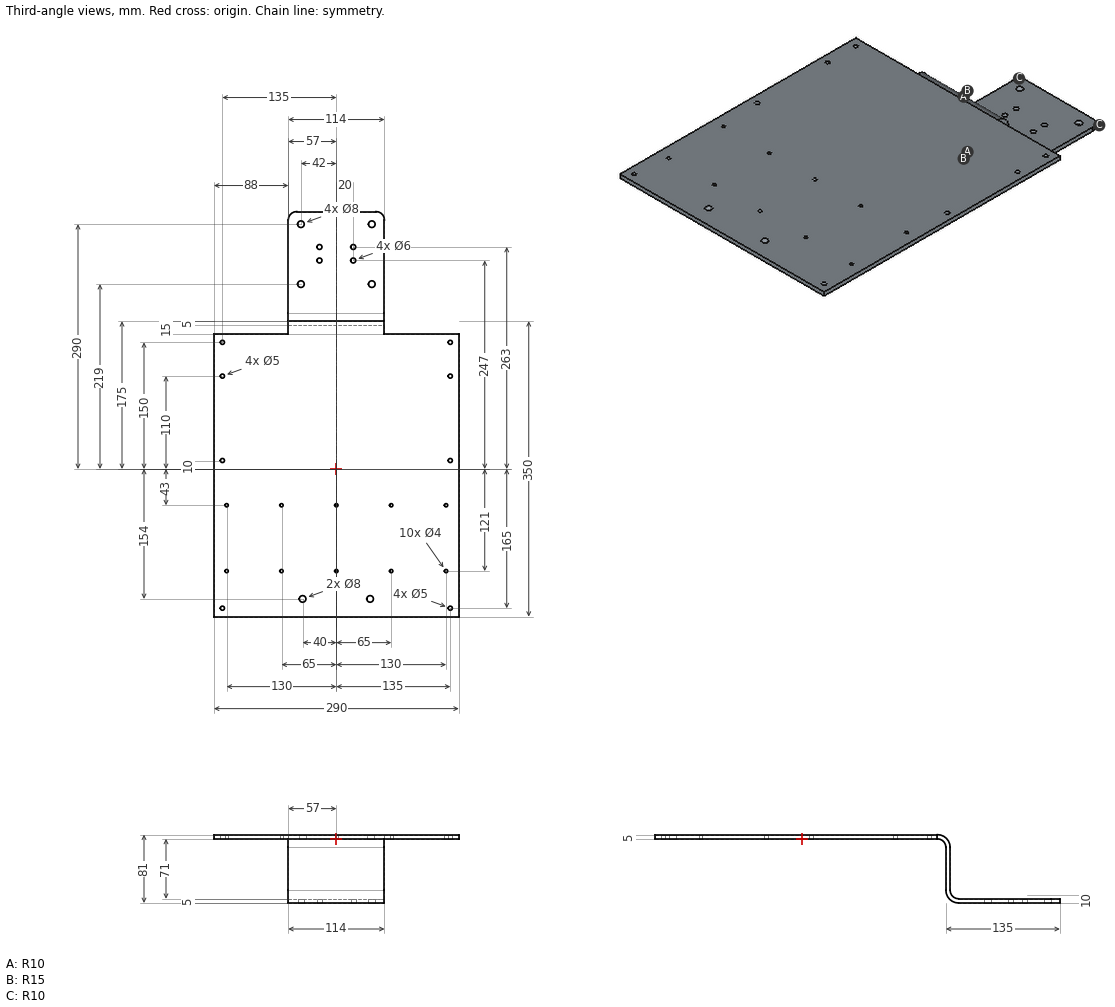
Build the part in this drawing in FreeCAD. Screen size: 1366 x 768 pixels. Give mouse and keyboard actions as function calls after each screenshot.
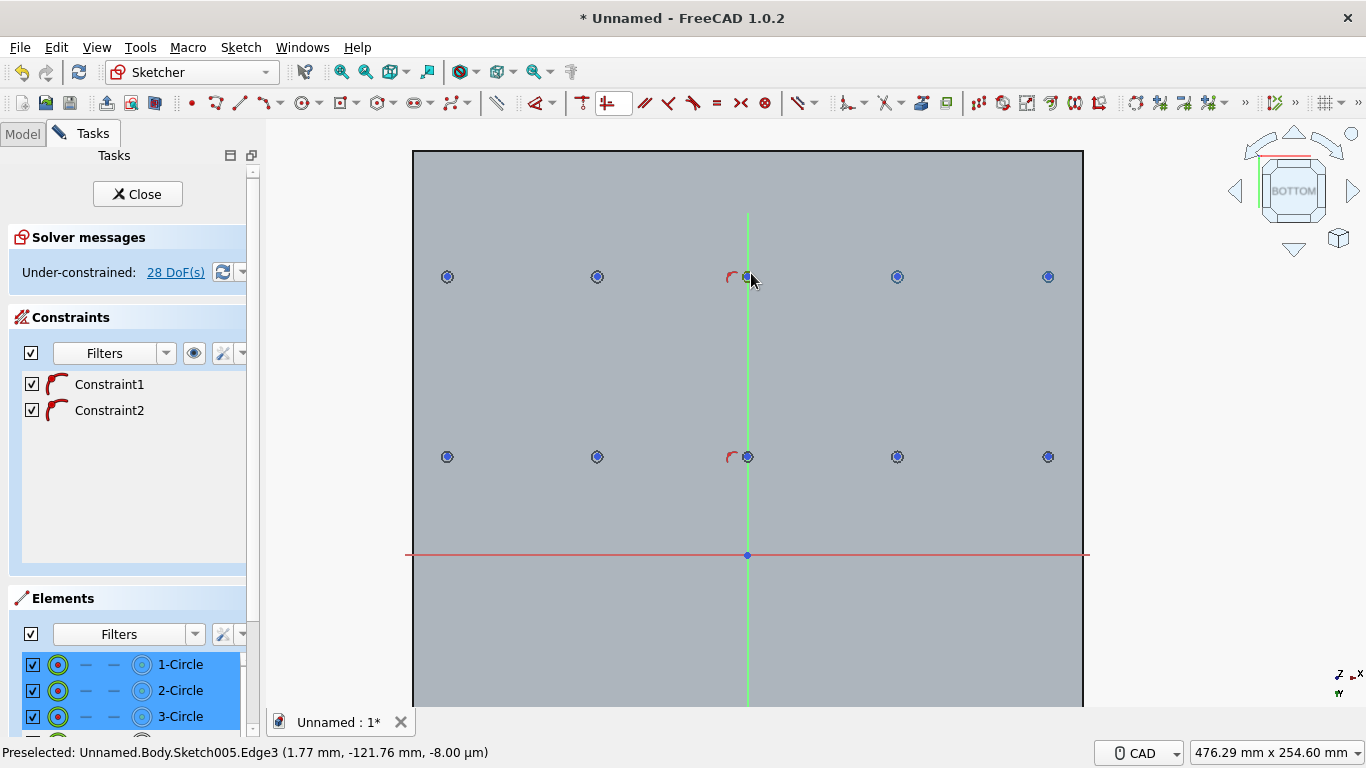
scroll(601, 273, up, 5)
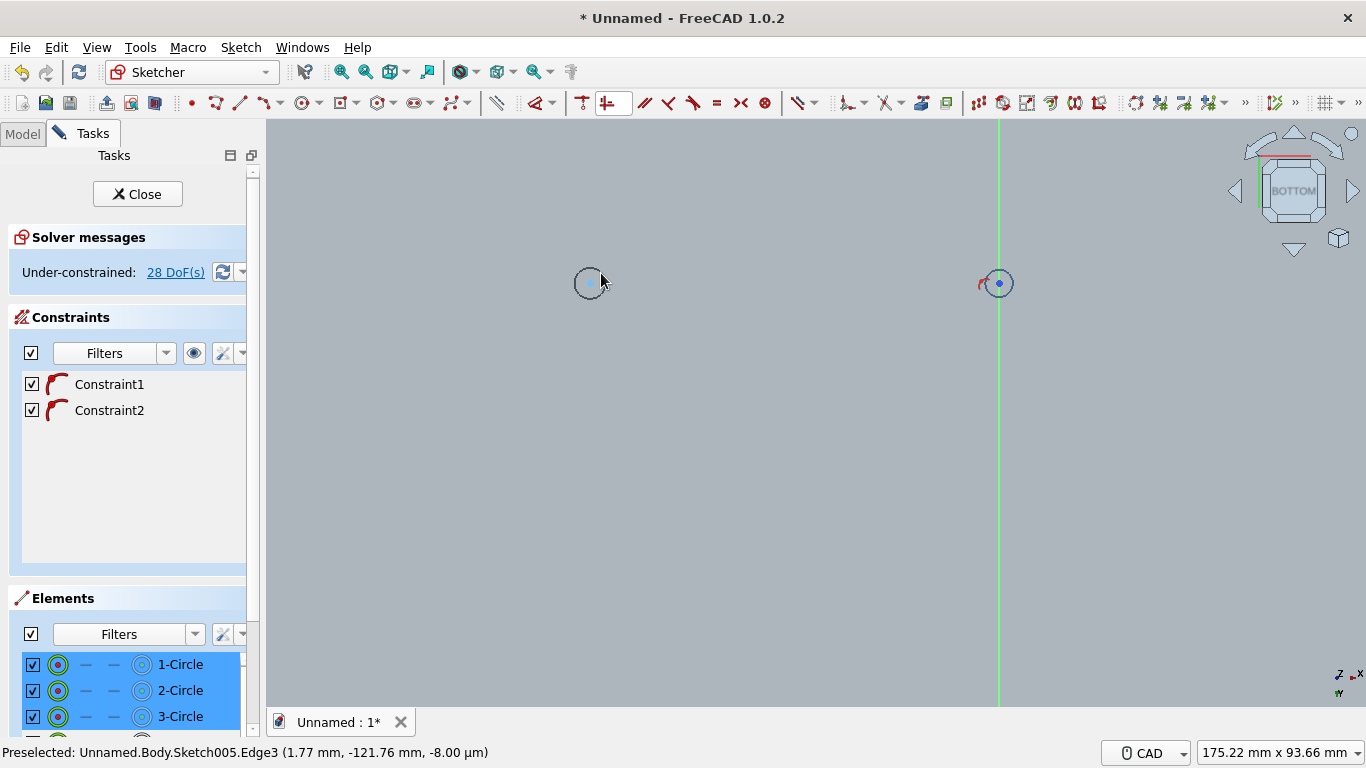
click(601, 272)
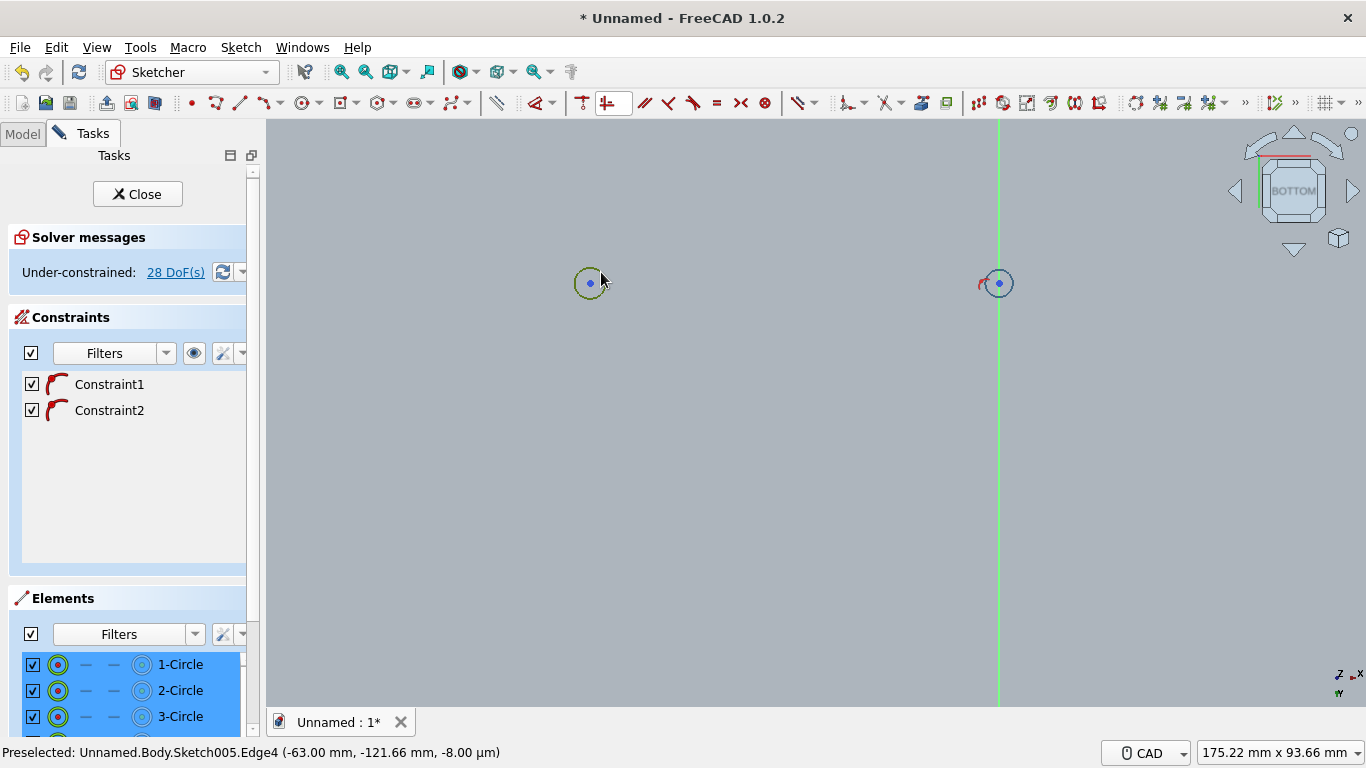
scroll(601, 273, down, 5)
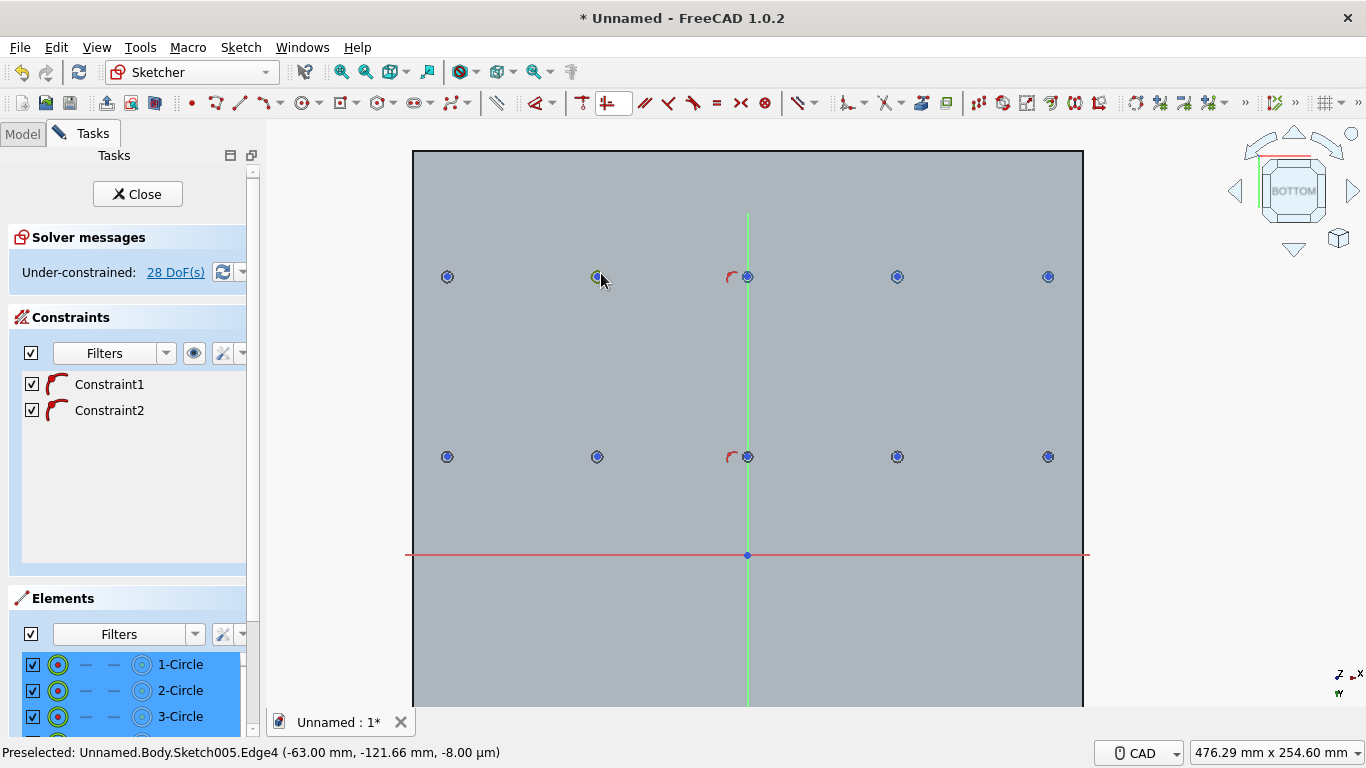
scroll(451, 273, up, 5)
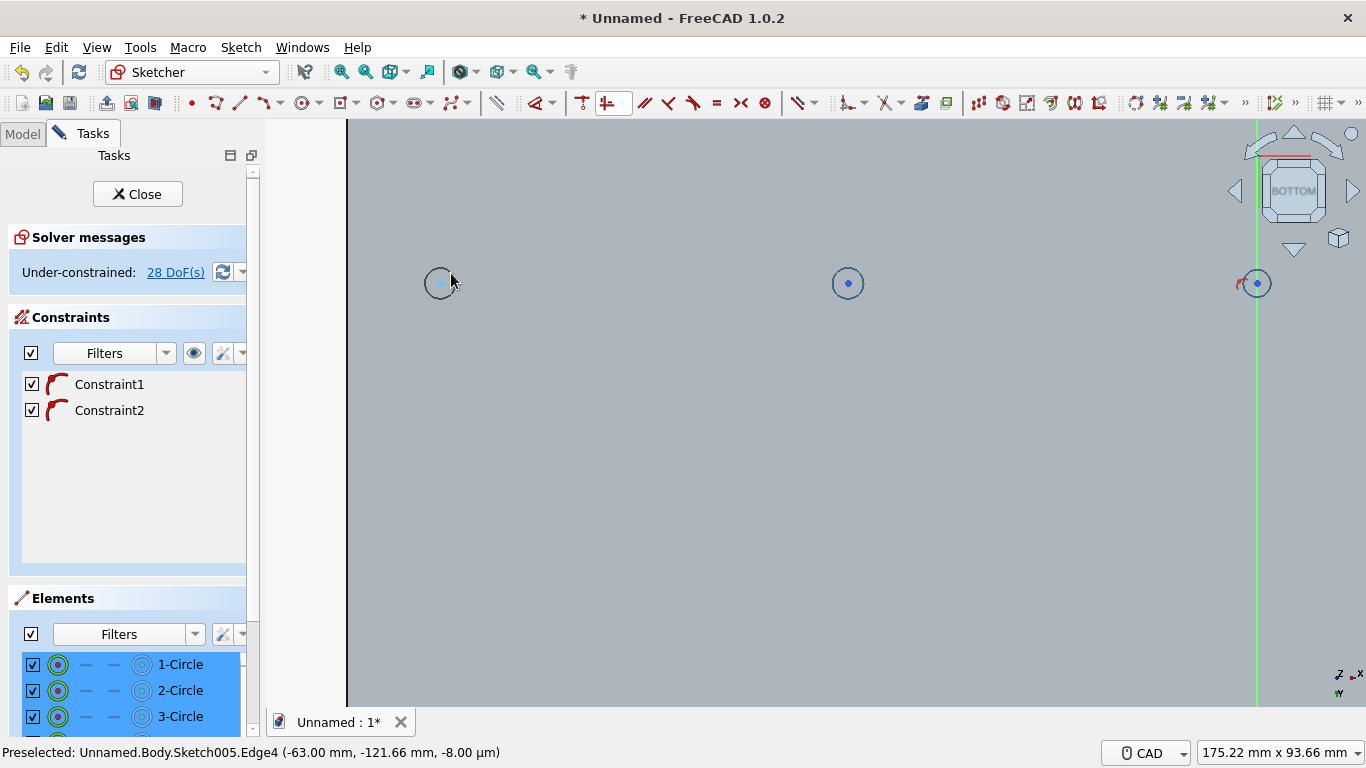
click(451, 273)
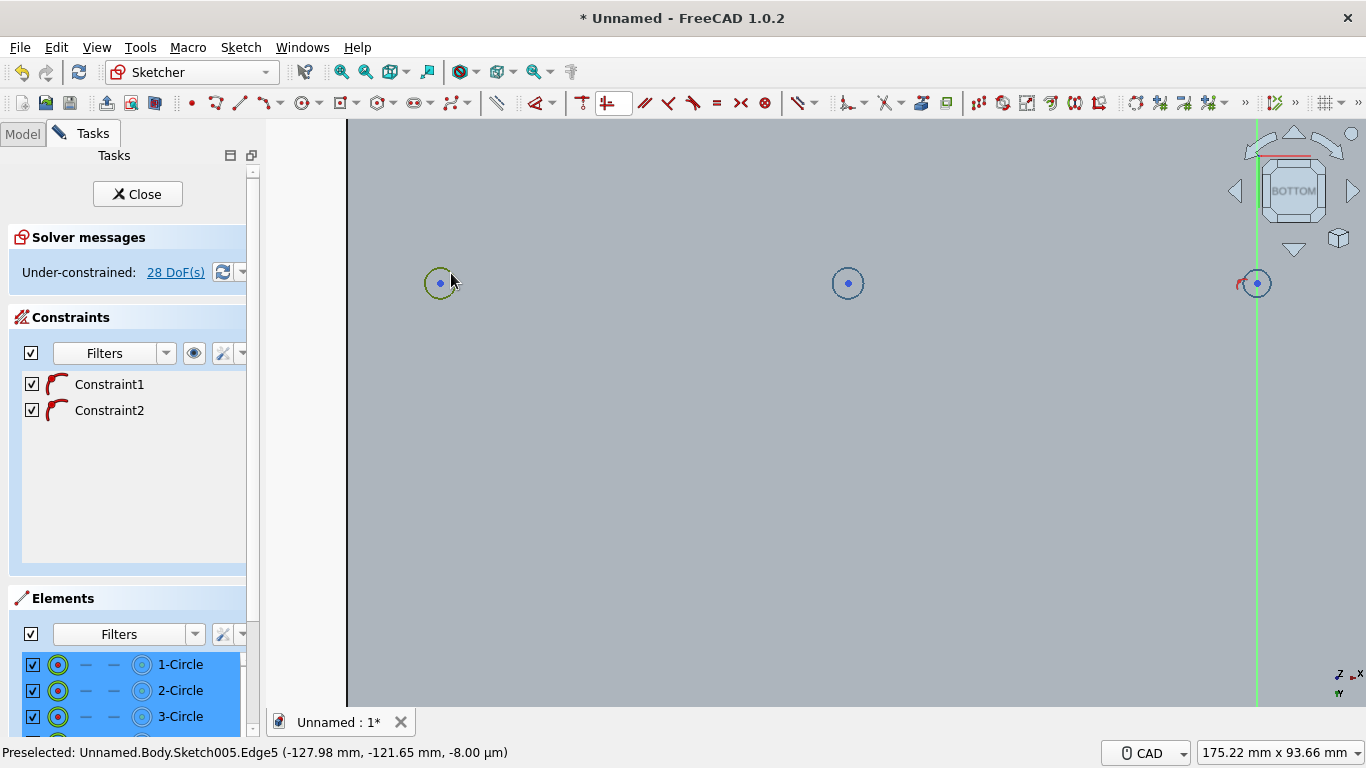
scroll(451, 273, down, 5)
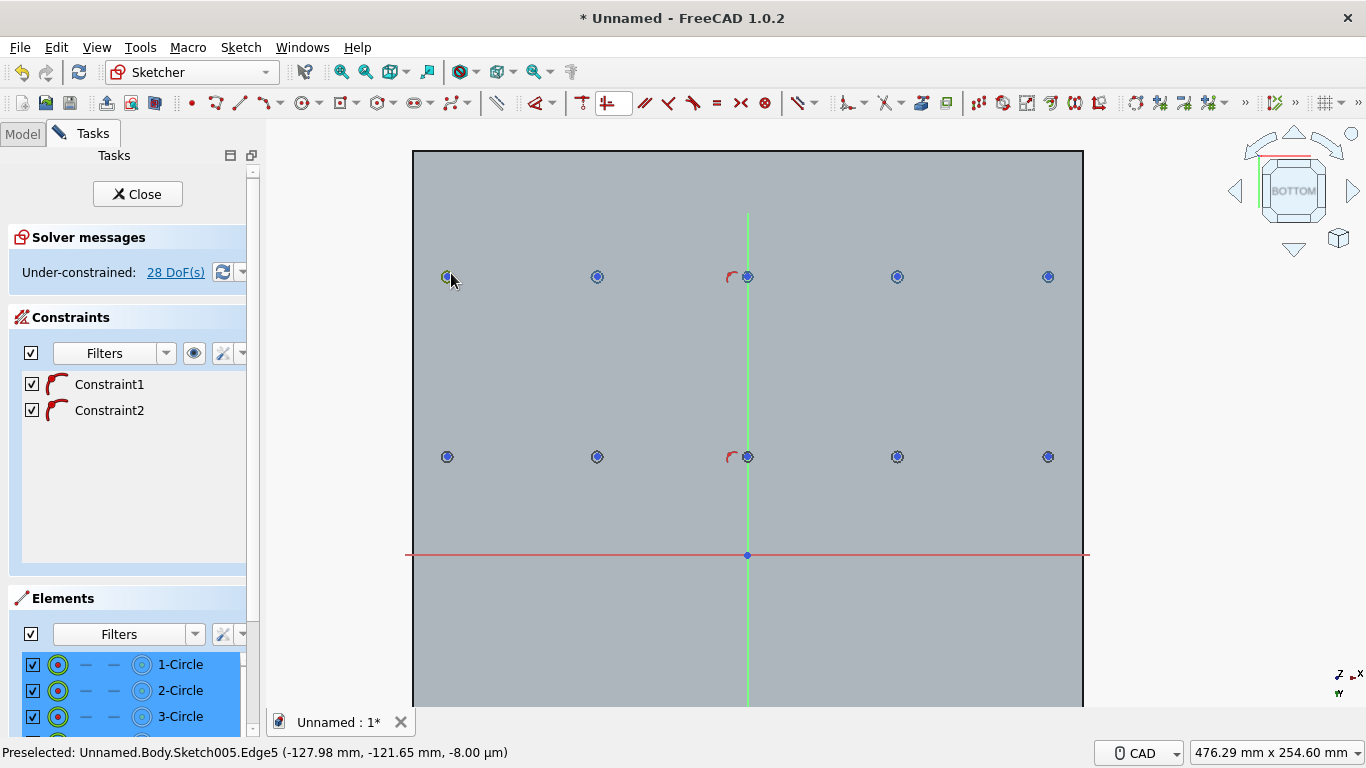
scroll(451, 453, up, 5)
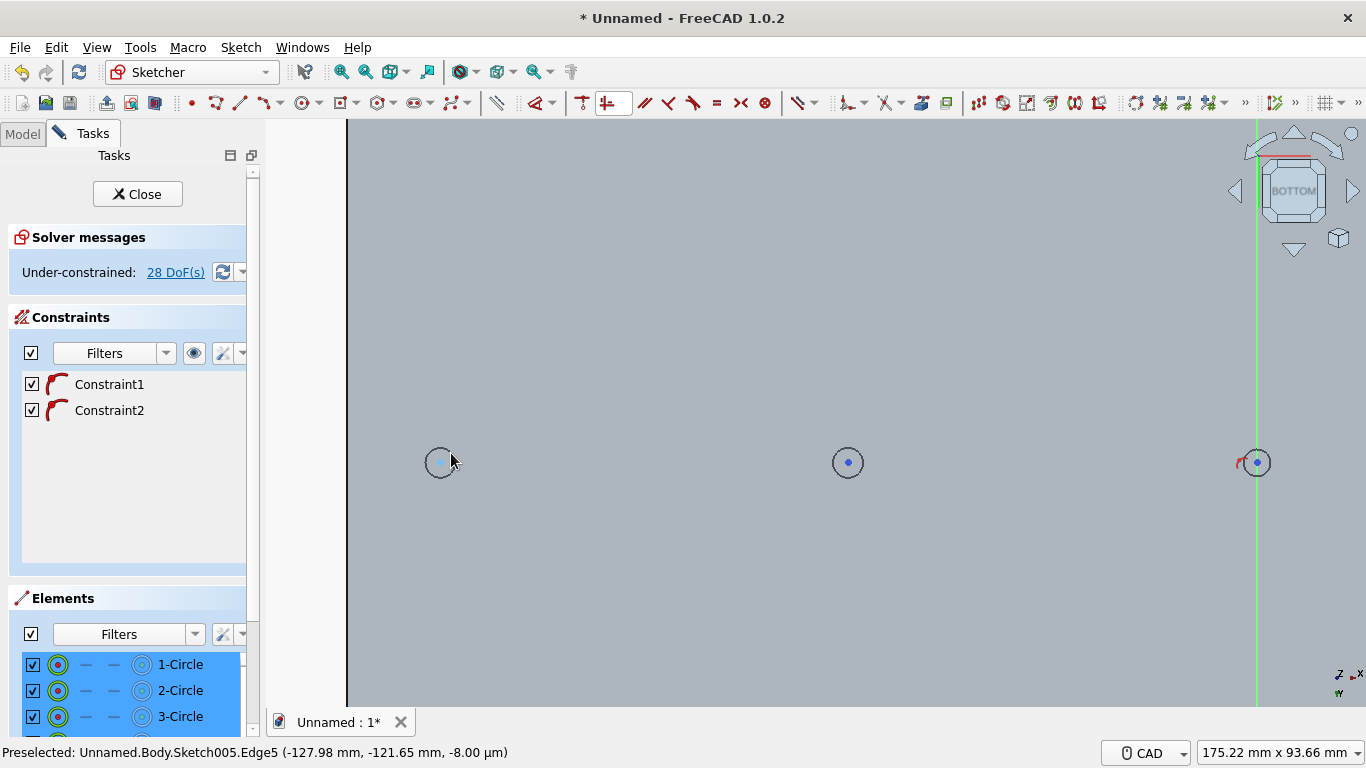
click(451, 452)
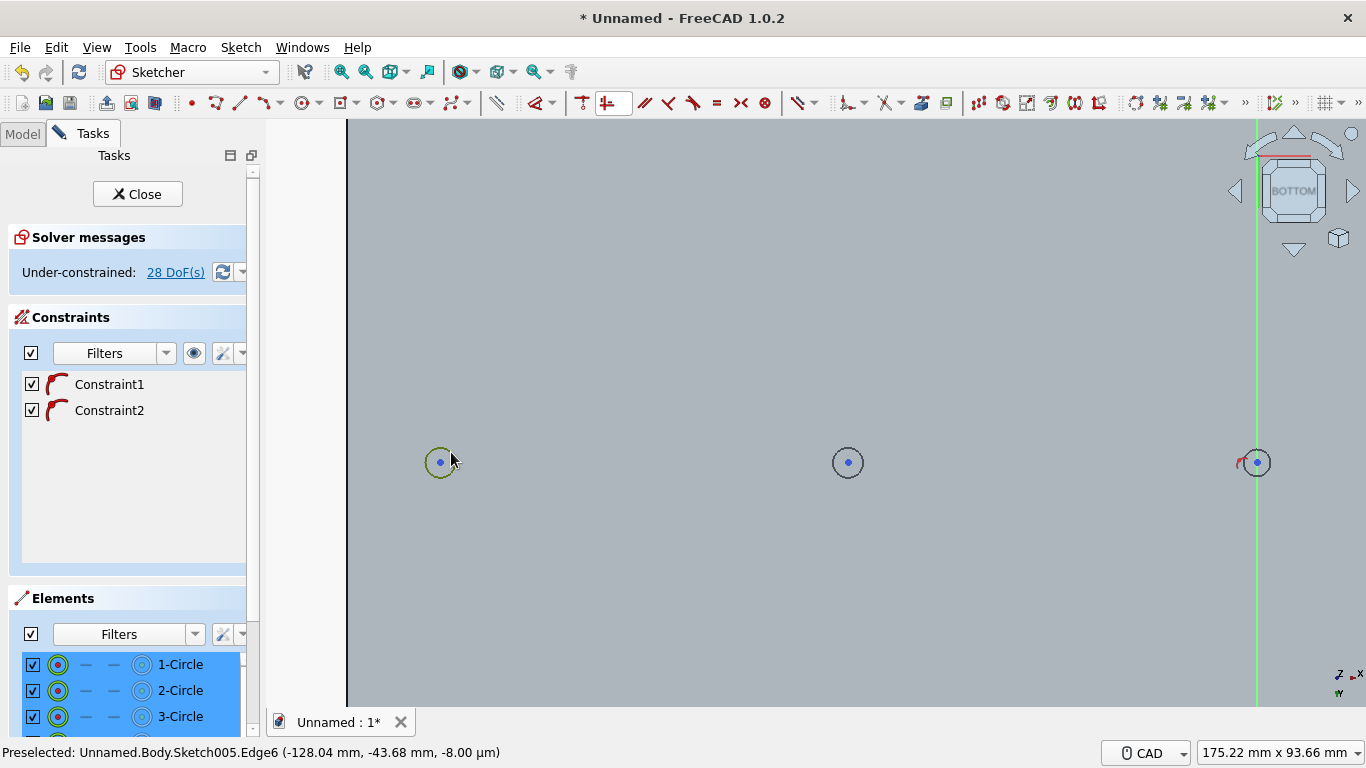
click(859, 452)